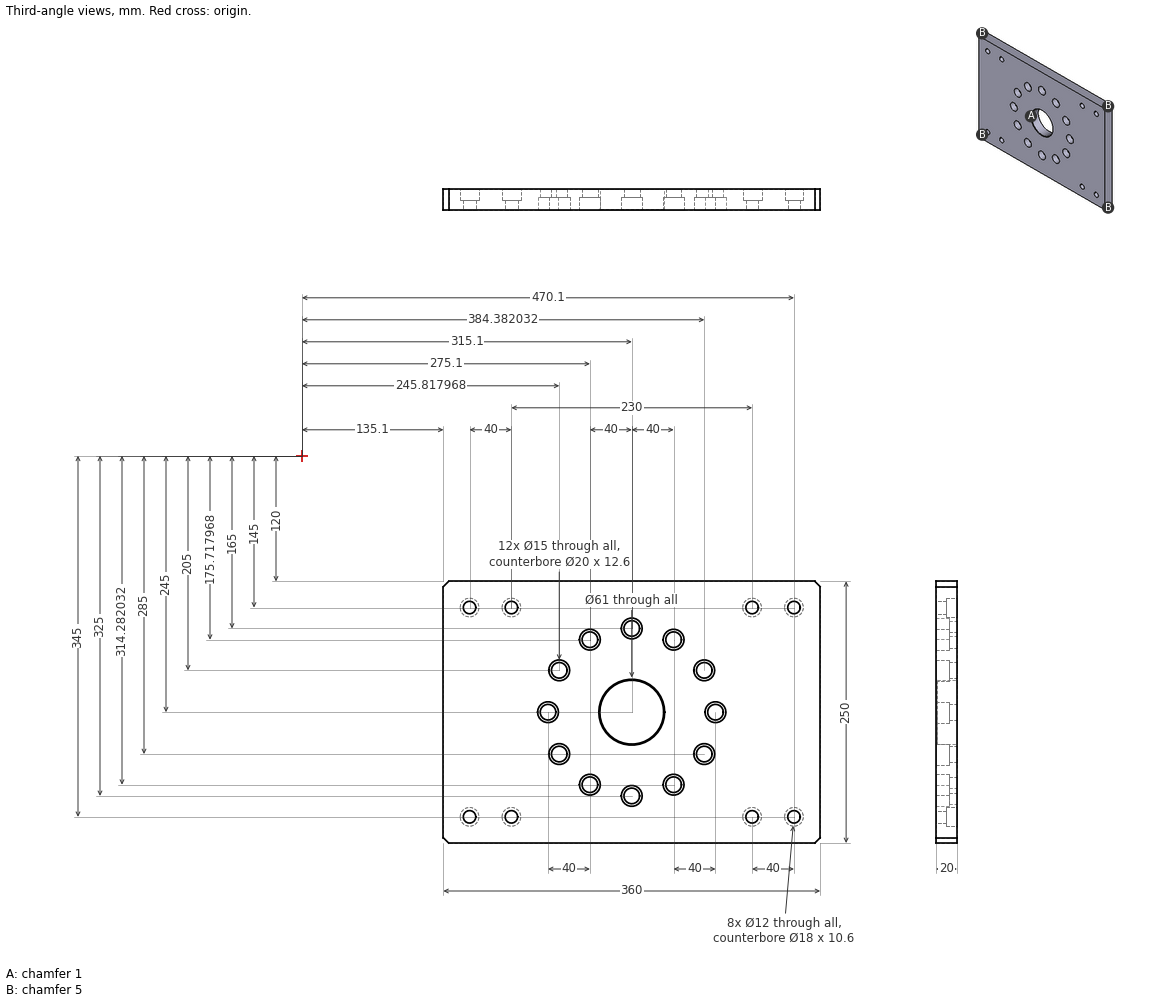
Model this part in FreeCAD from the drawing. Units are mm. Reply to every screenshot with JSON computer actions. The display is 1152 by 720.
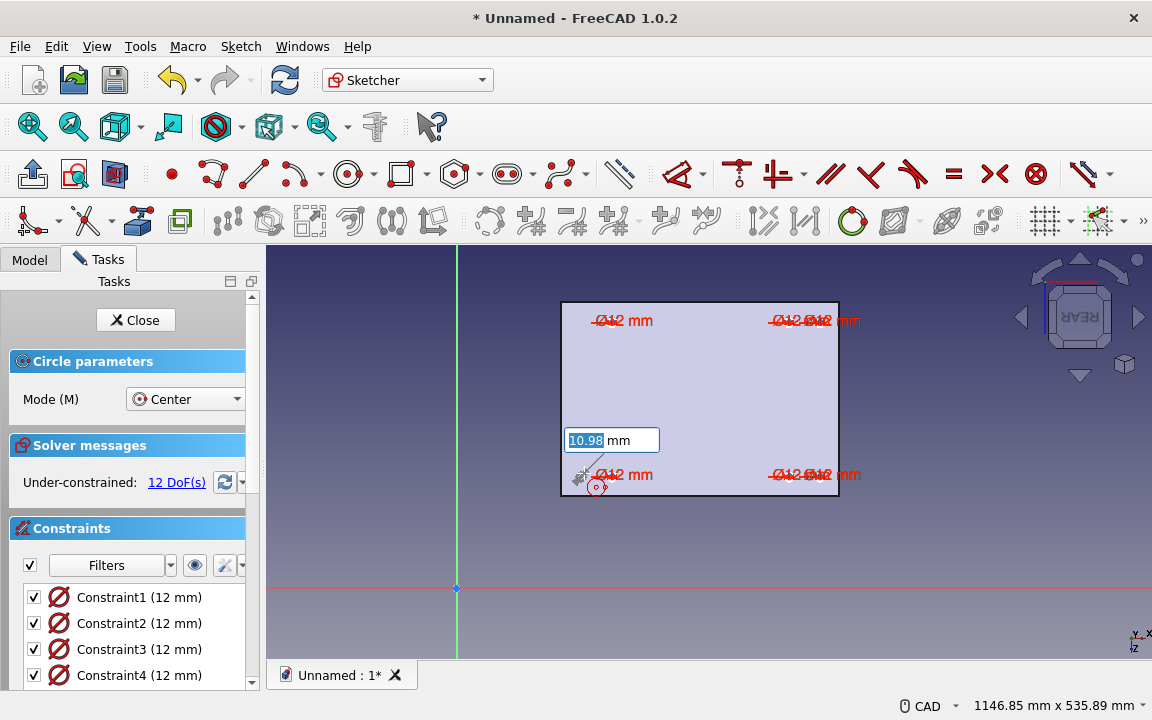
{"action": "type", "text": "12"}
{"action": "key", "text": "Return"}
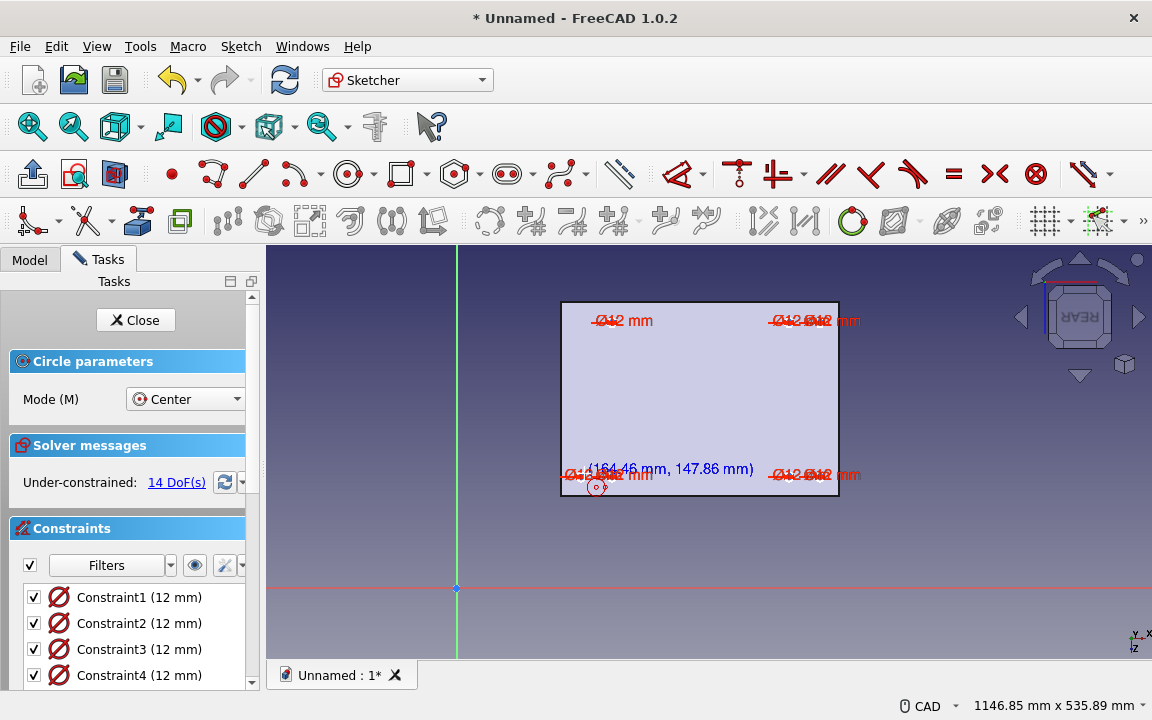
{"action": "scroll", "coordinate": [581, 322], "scroll_direction": "up", "scroll_amount": 8}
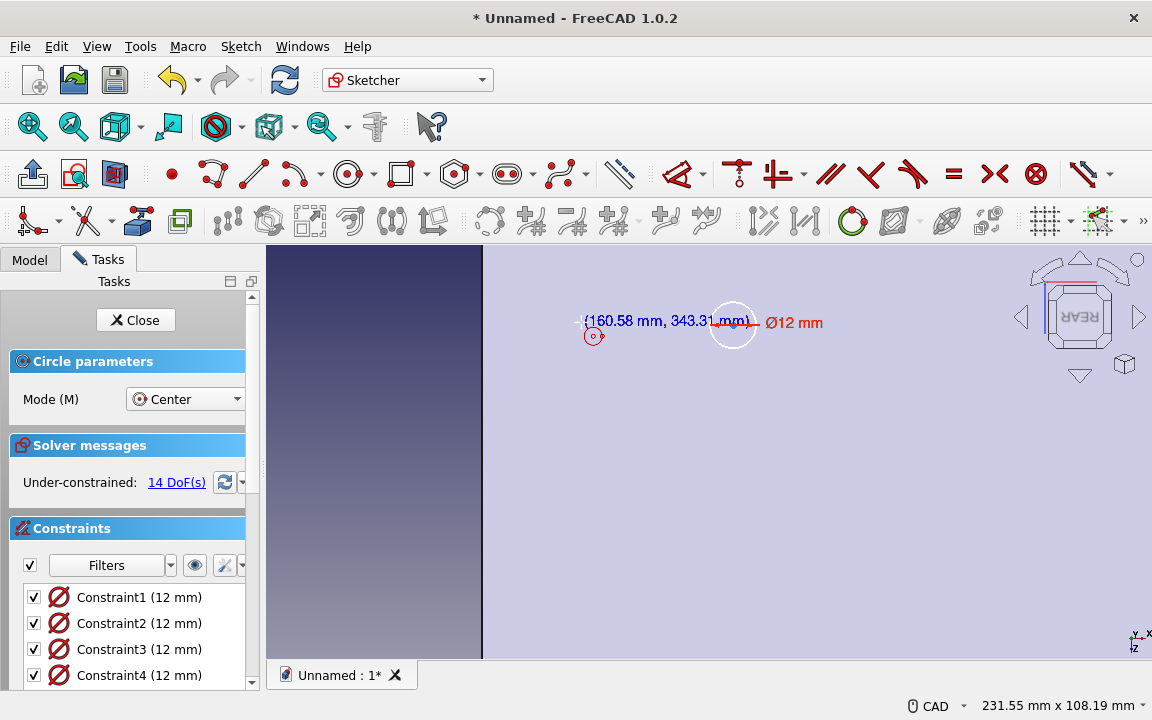
{"action": "scroll", "coordinate": [581, 321], "scroll_direction": "down", "scroll_amount": 8}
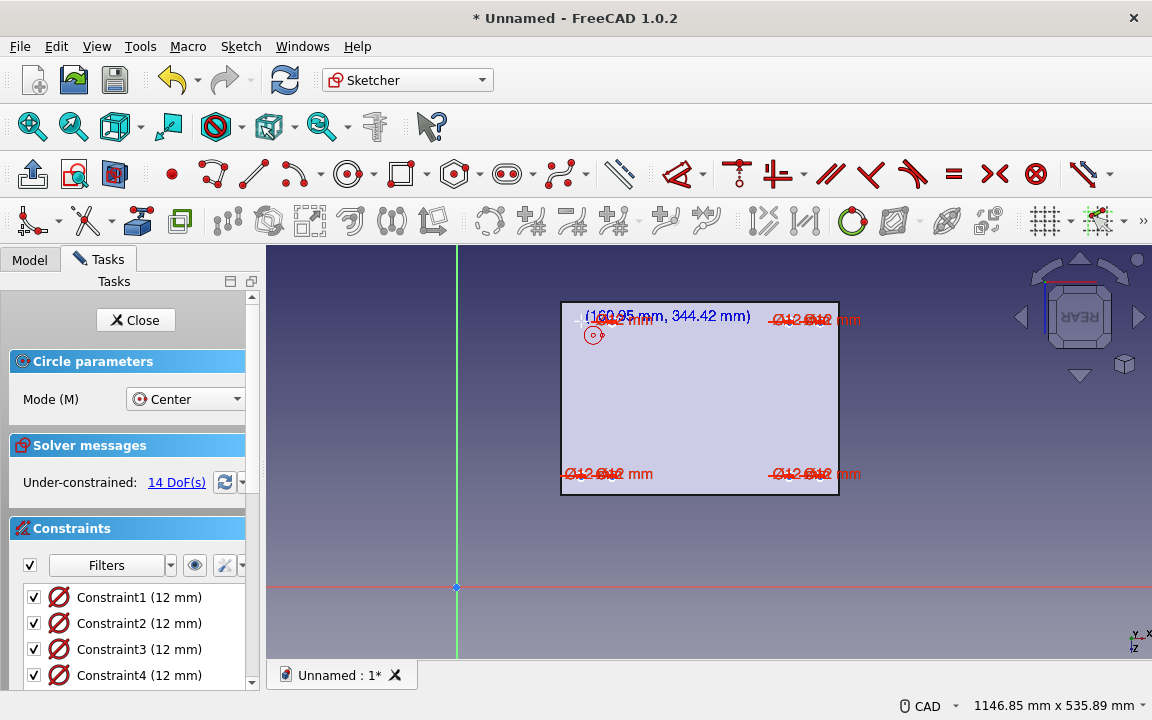
{"action": "left_click", "coordinate": [581, 321]}
{"action": "mouse_move", "coordinate": [584, 318]}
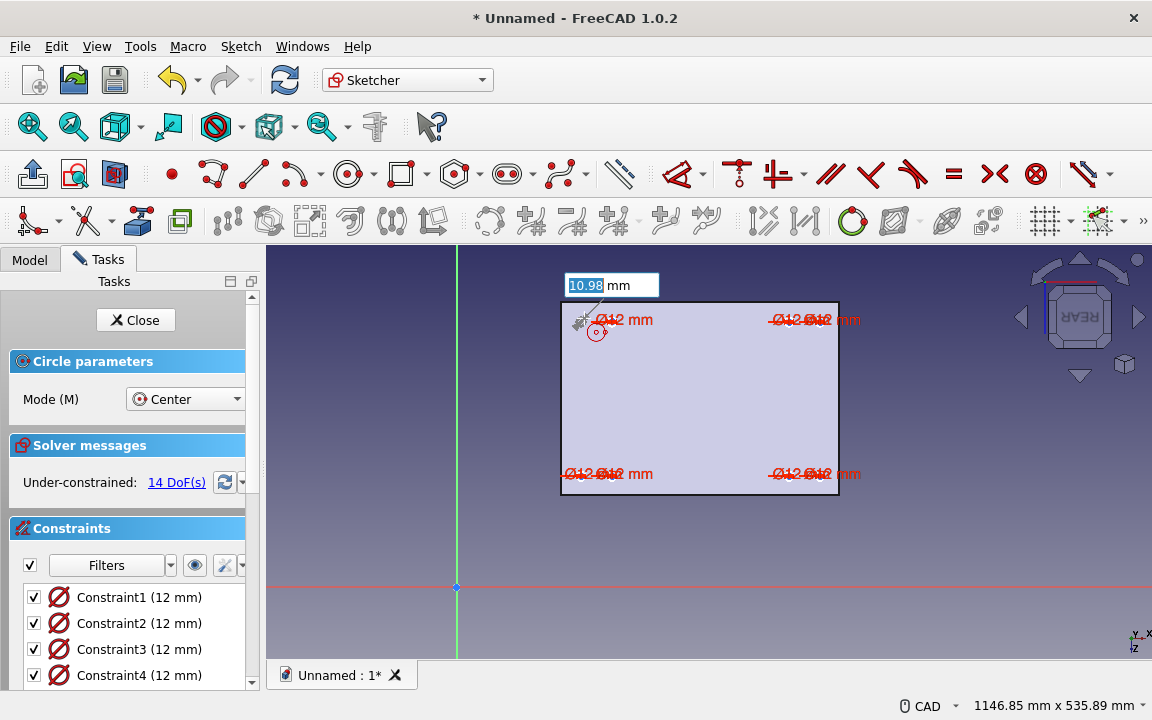
{"action": "type", "text": "12"}
{"action": "key", "text": "Return"}
{"action": "key", "text": "Escape"}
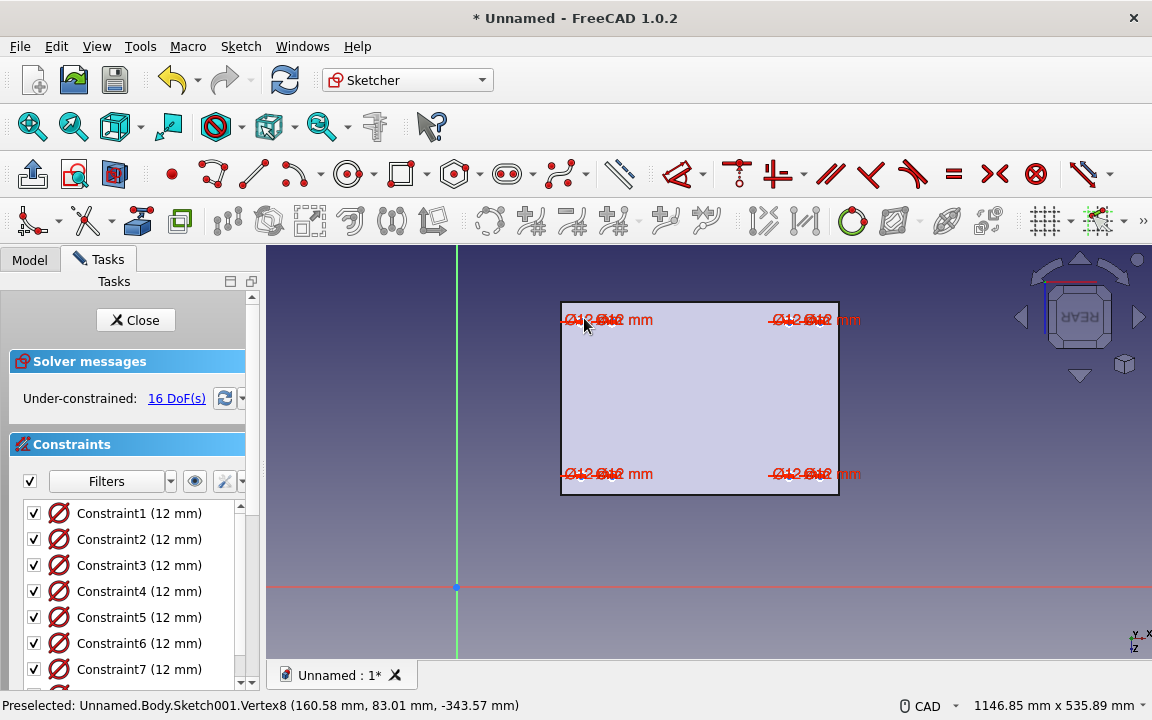
{"action": "left_click", "coordinate": [676, 174]}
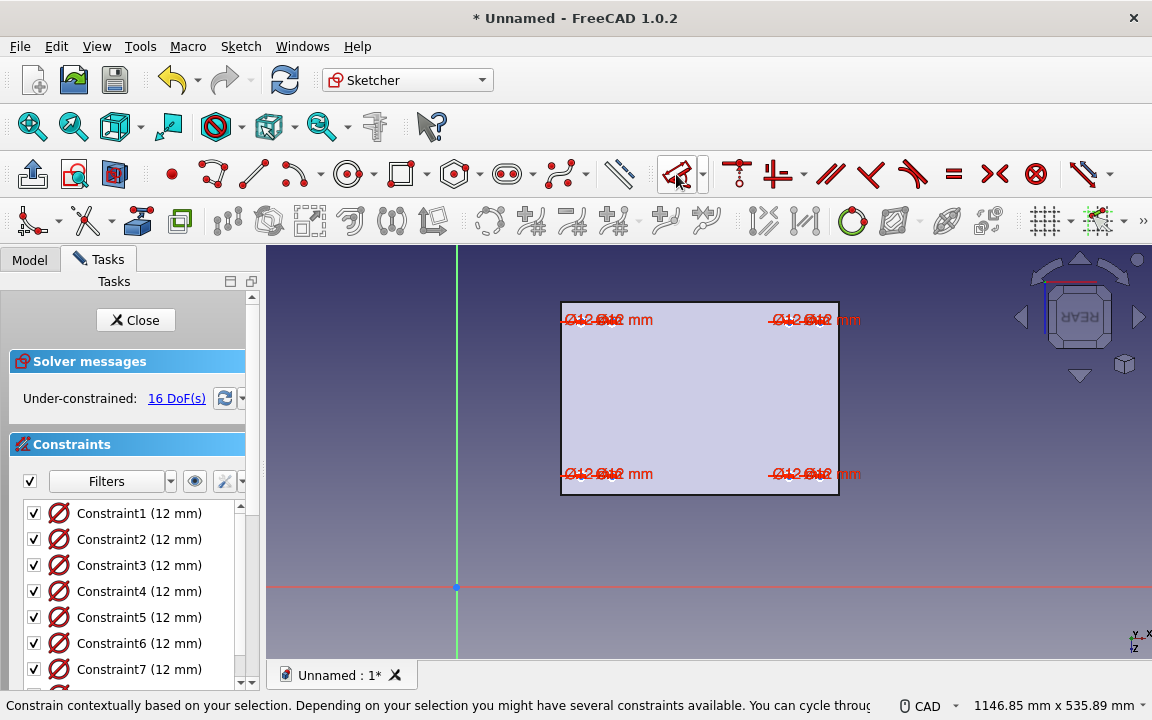
{"action": "left_click", "coordinate": [820, 322]}
{"action": "left_click", "coordinate": [423, 455]}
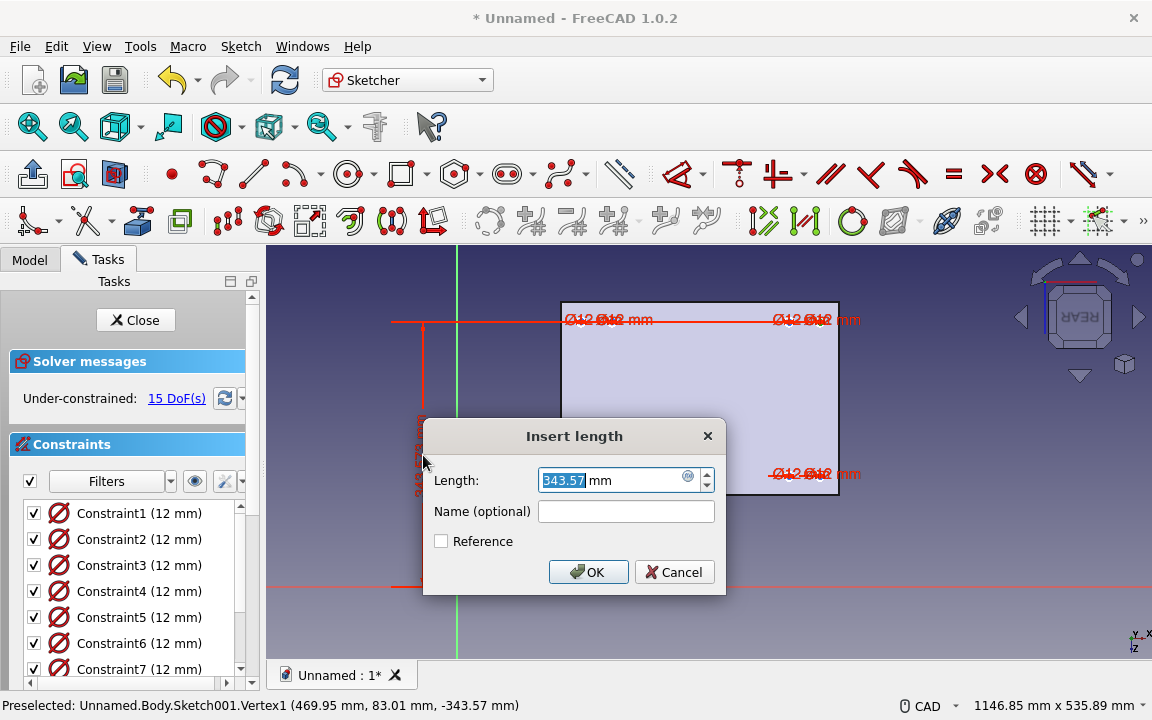
{"action": "type", "text": "345"}
{"action": "key", "text": "Return"}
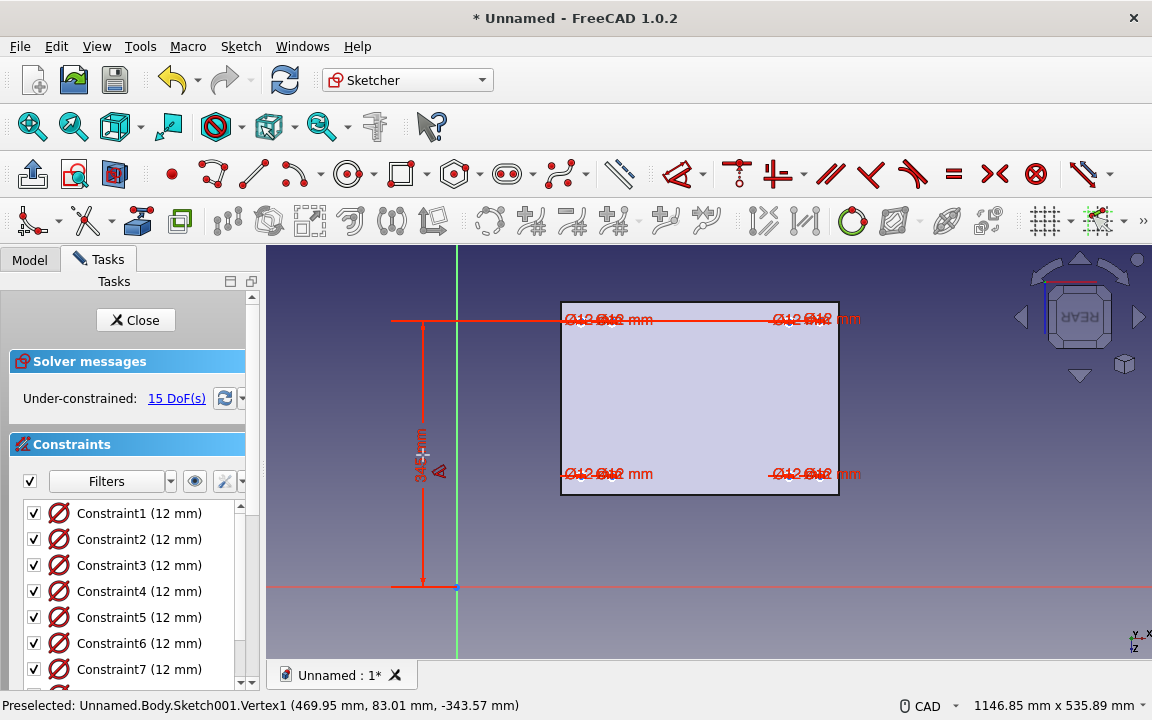
{"action": "left_click", "coordinate": [789, 322]}
{"action": "left_click", "coordinate": [423, 394]}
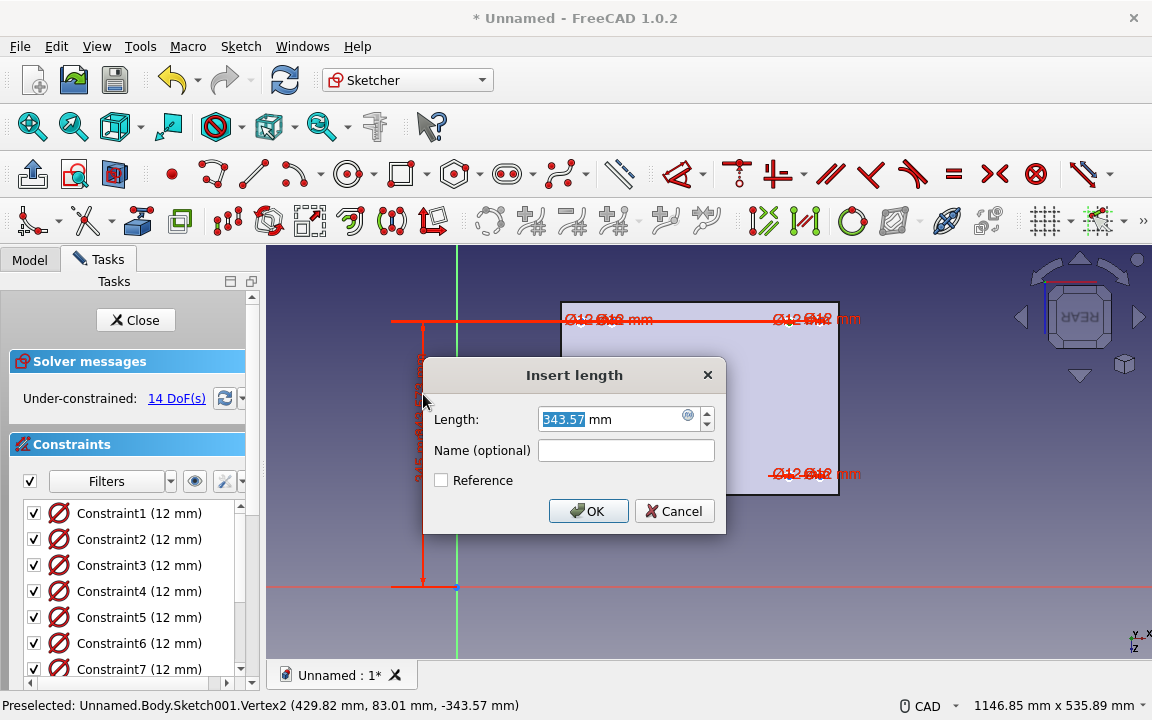
{"action": "type", "text": "345"}
{"action": "key", "text": "Return"}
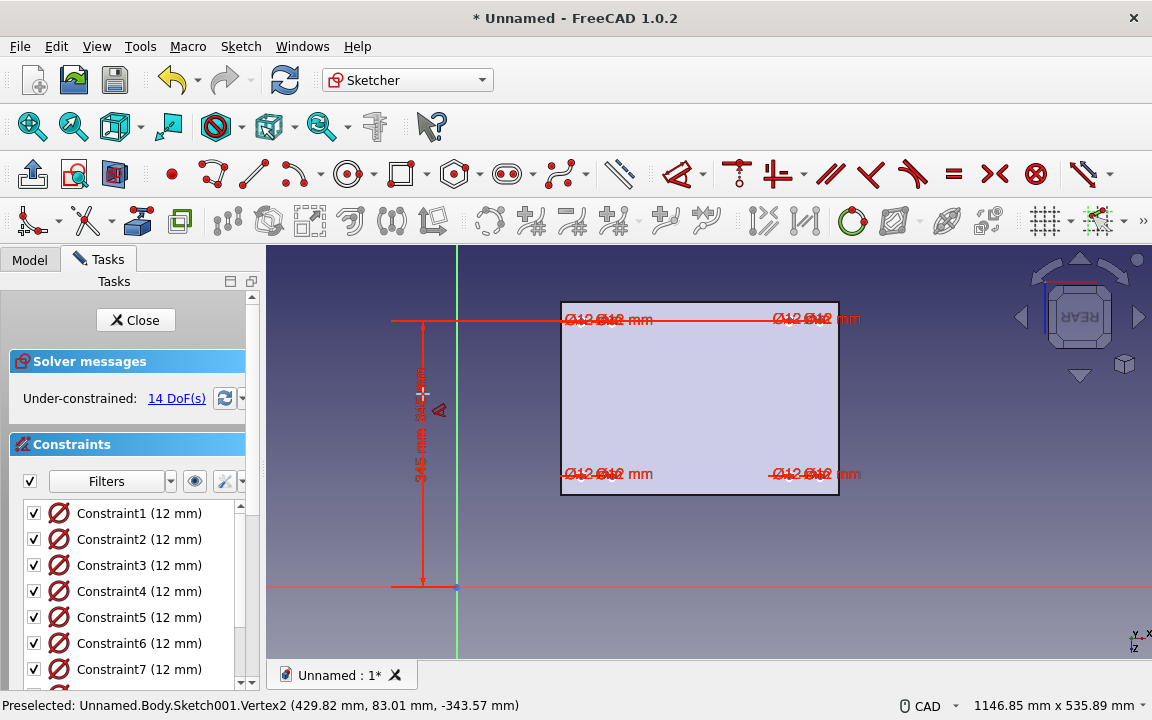
{"action": "left_click", "coordinate": [820, 476]}
{"action": "left_click", "coordinate": [423, 532]}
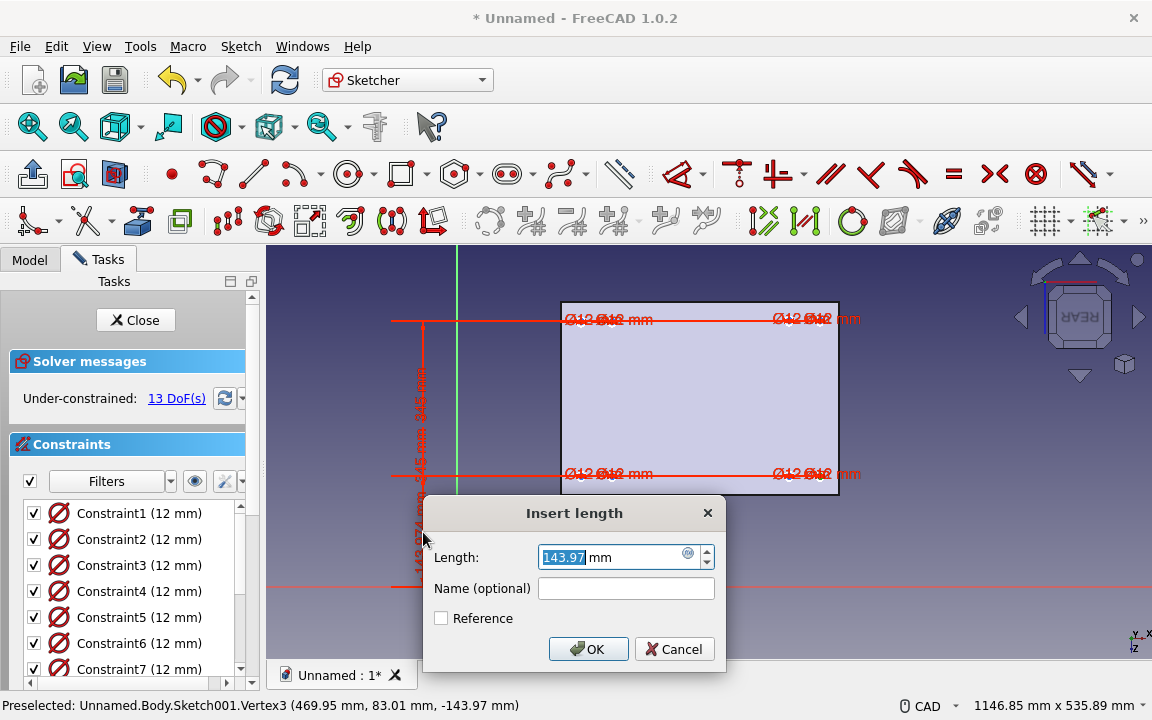
{"action": "type", "text": "145"}
{"action": "key", "text": "Return"}